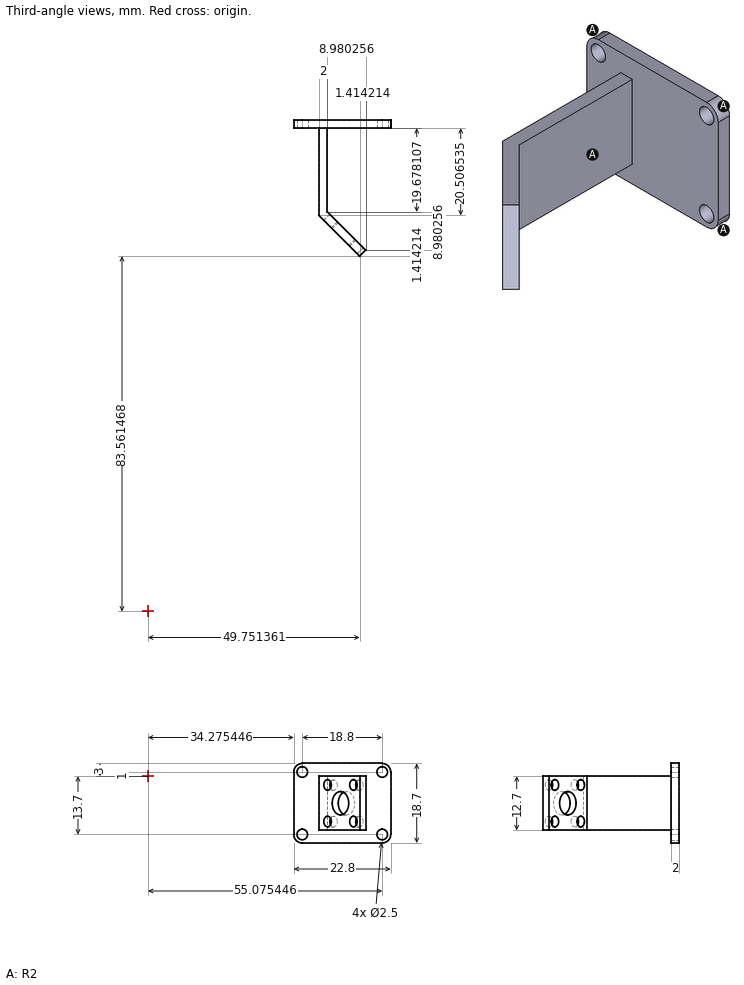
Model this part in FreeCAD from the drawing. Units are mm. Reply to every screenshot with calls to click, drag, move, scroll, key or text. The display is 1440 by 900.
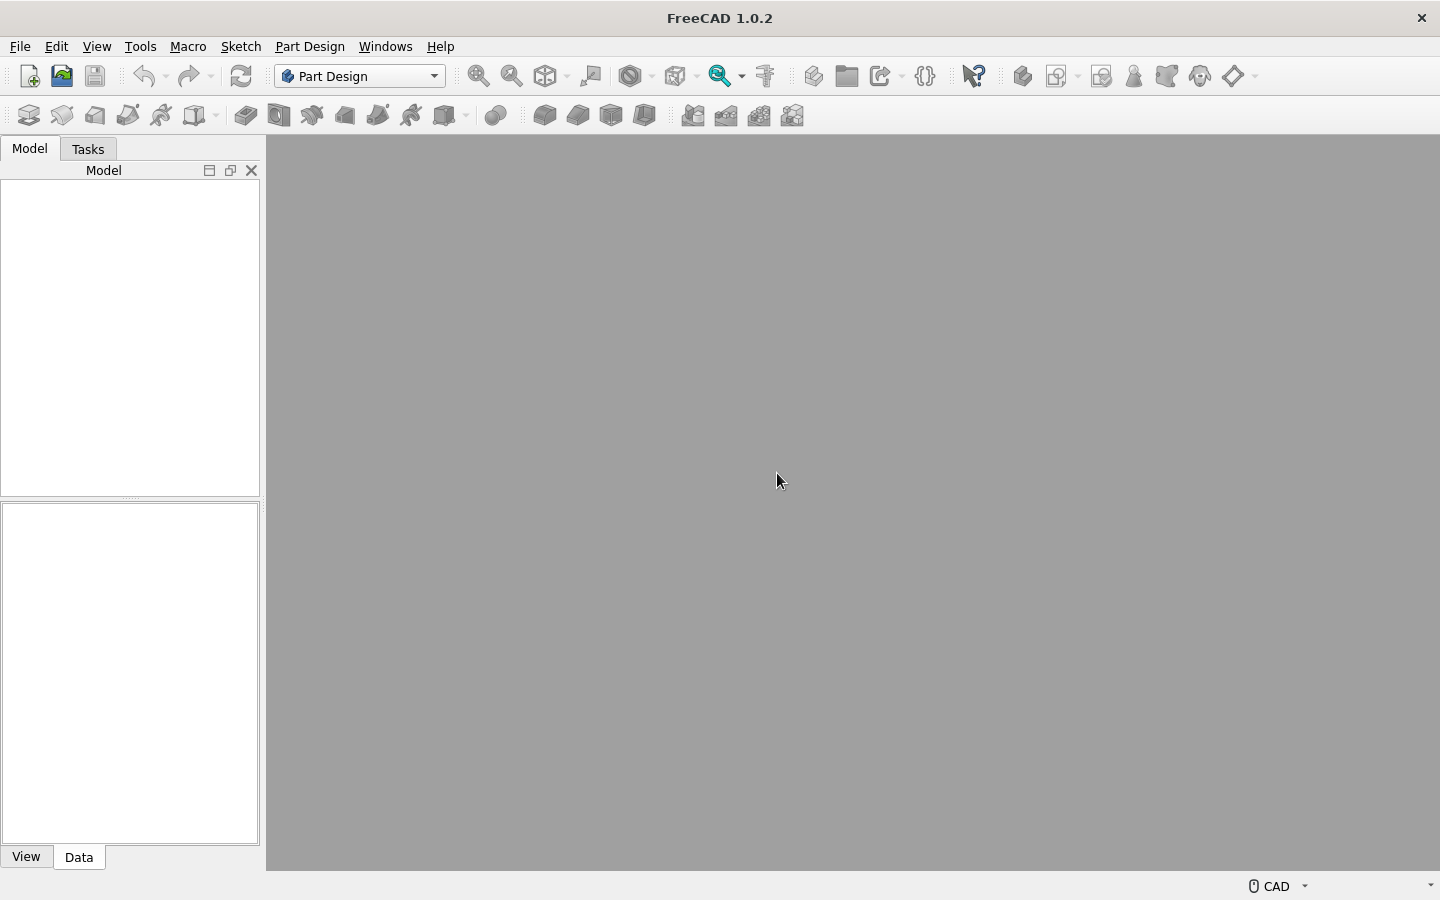
click(29, 76)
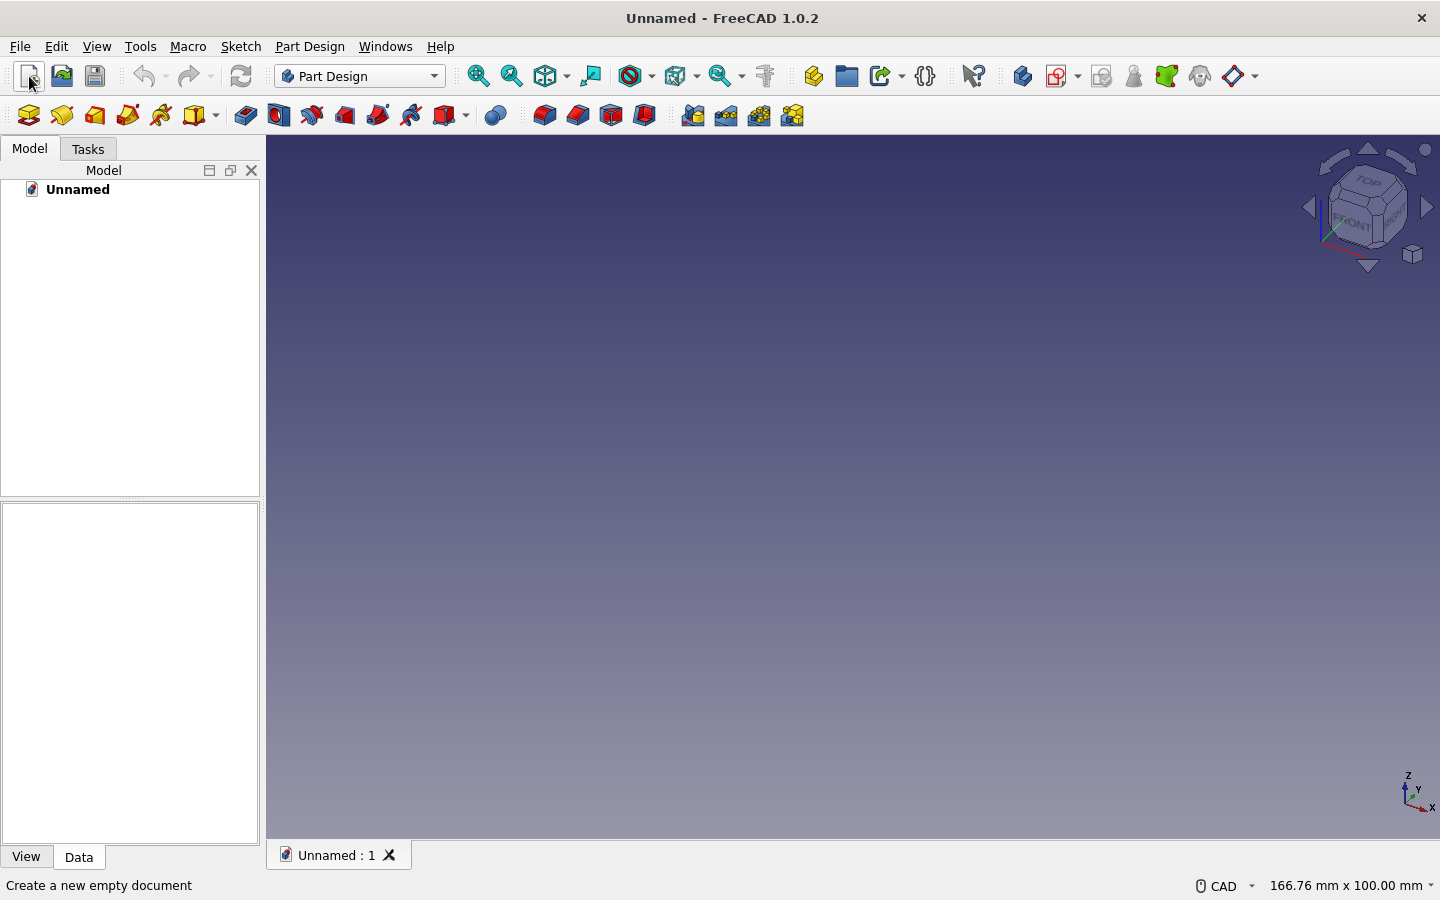
click(1056, 76)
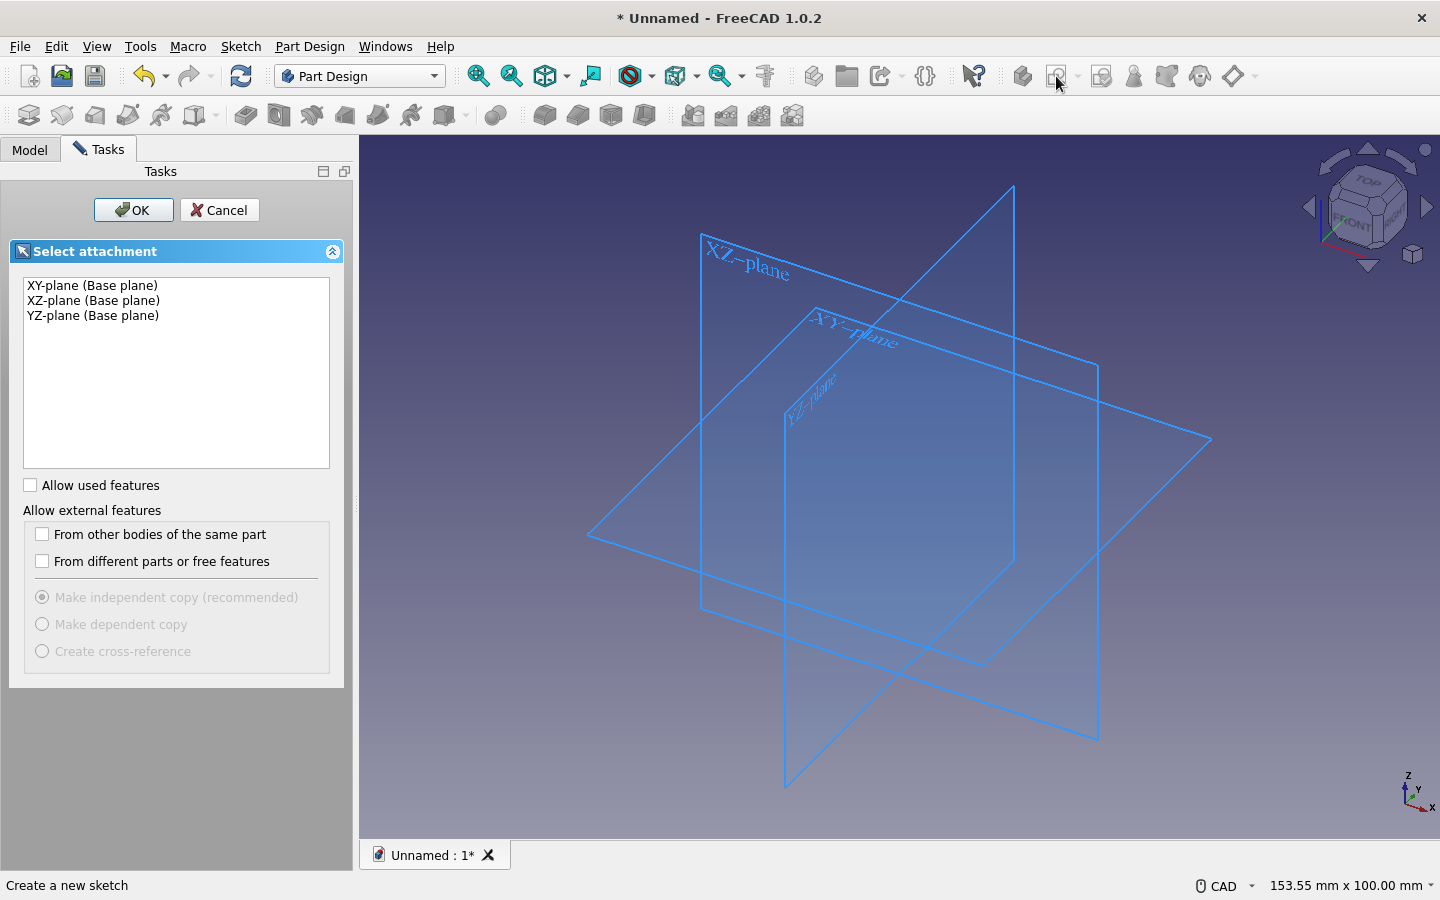
click(84, 286)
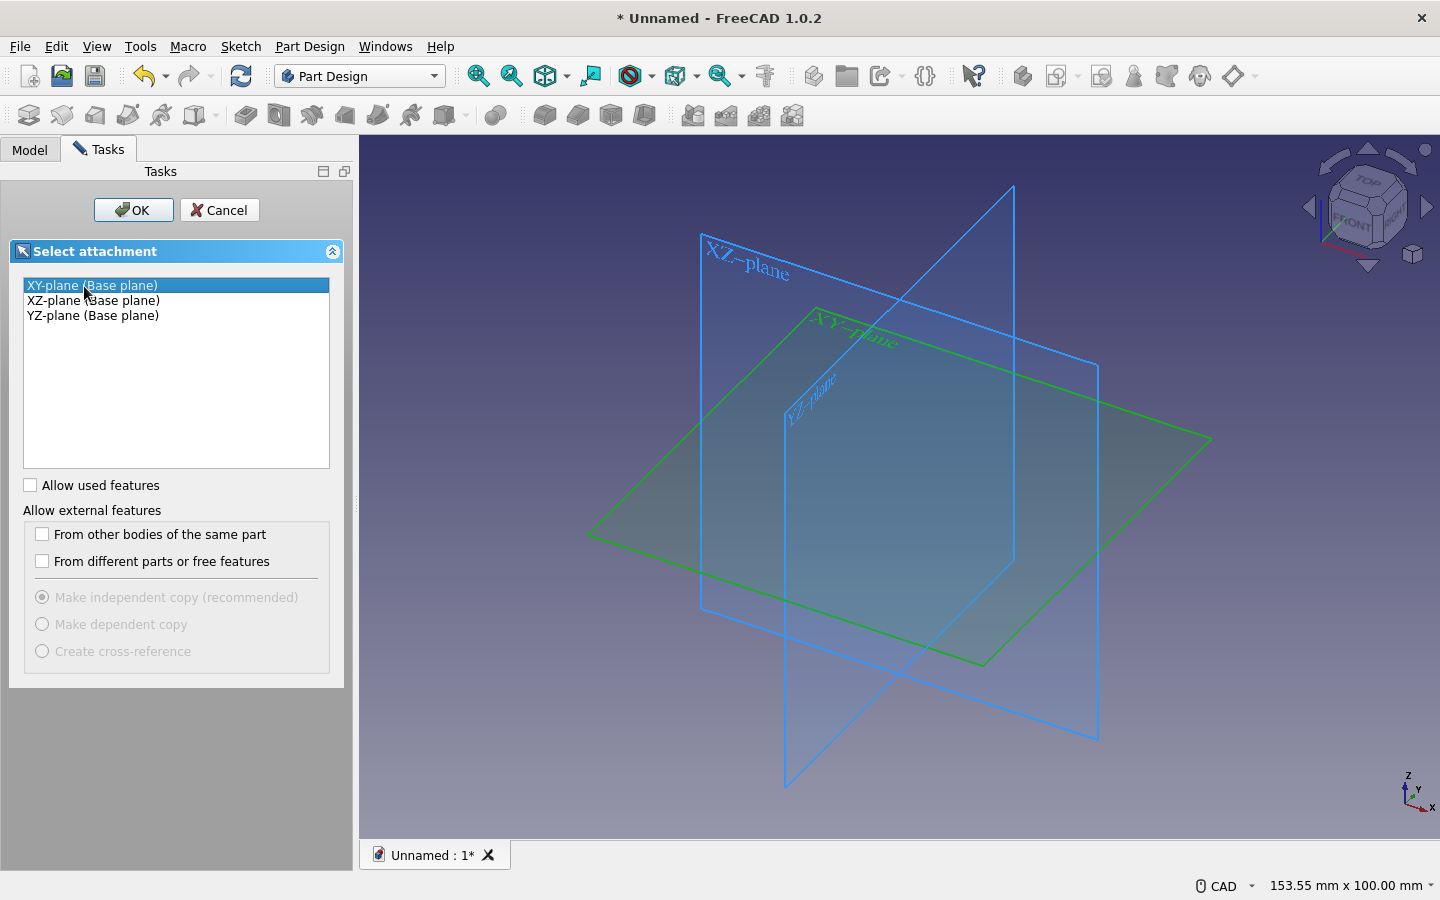
click(134, 210)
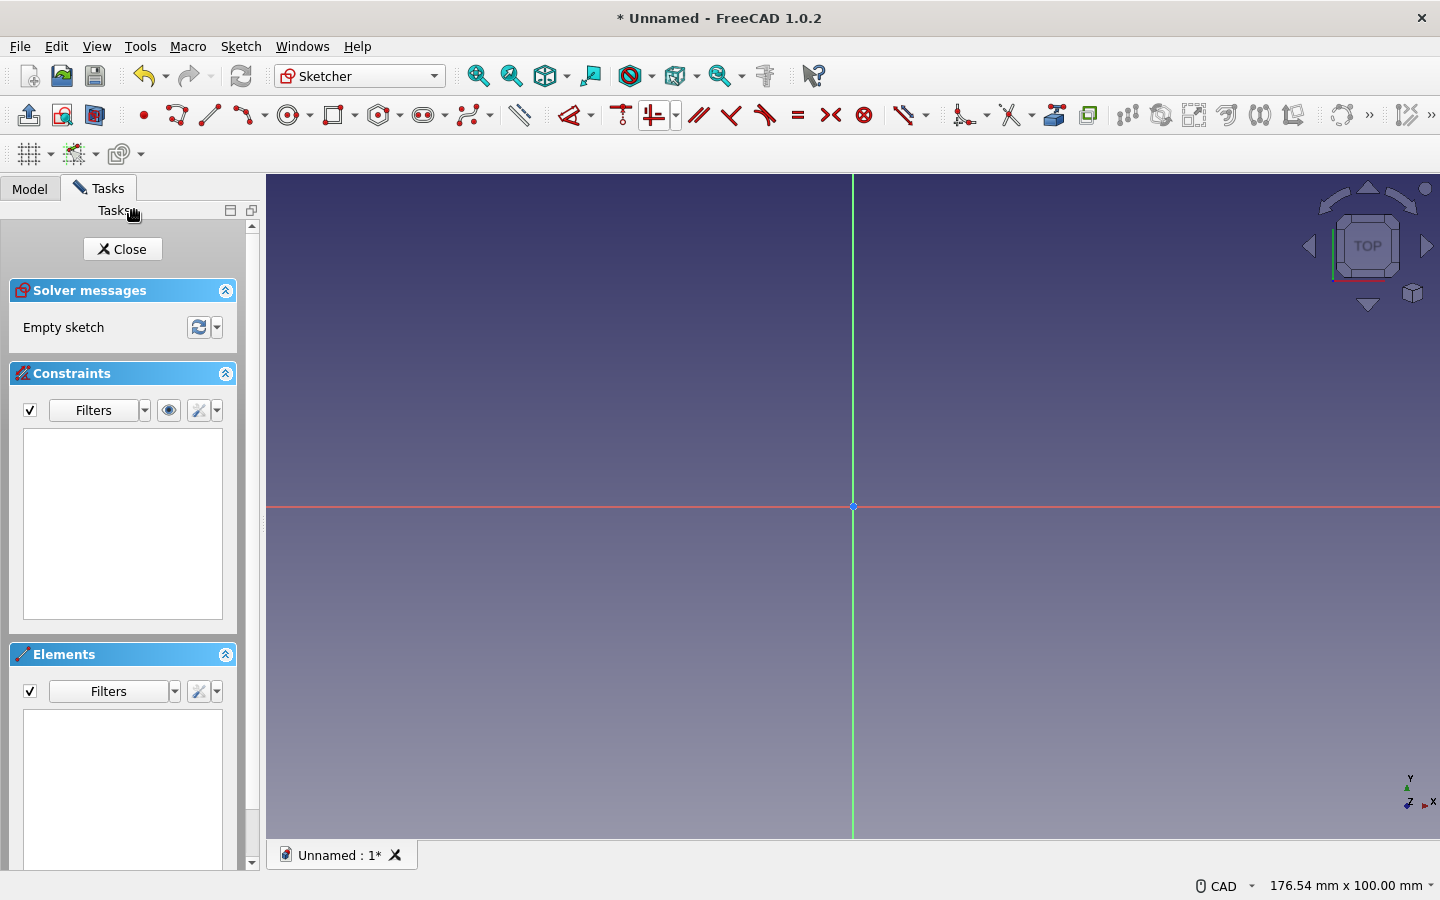
scroll(784, 506, down, 5)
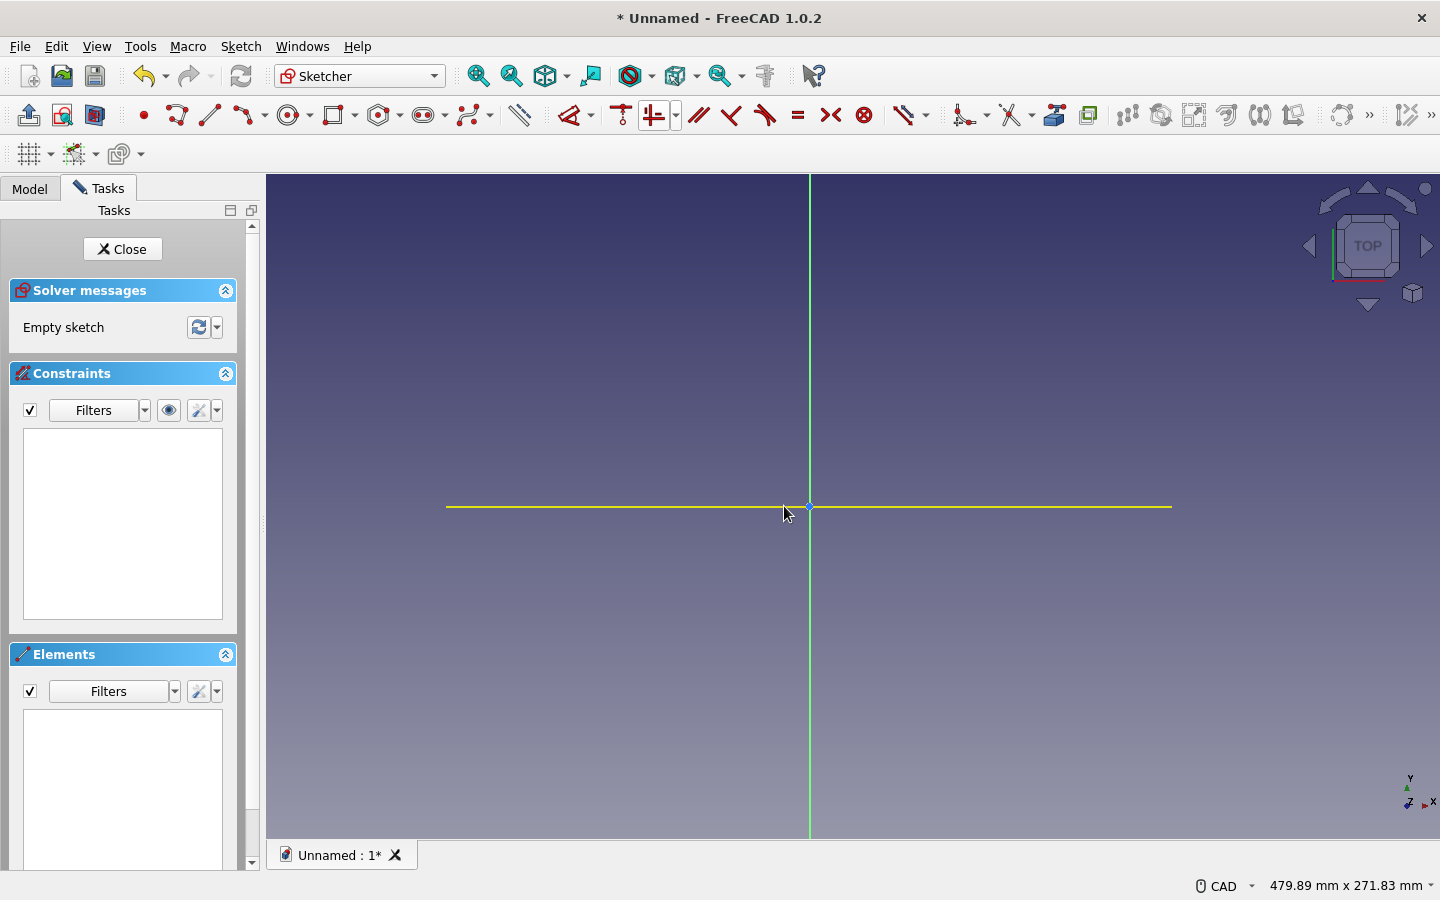
scroll(949, 218, up, 9)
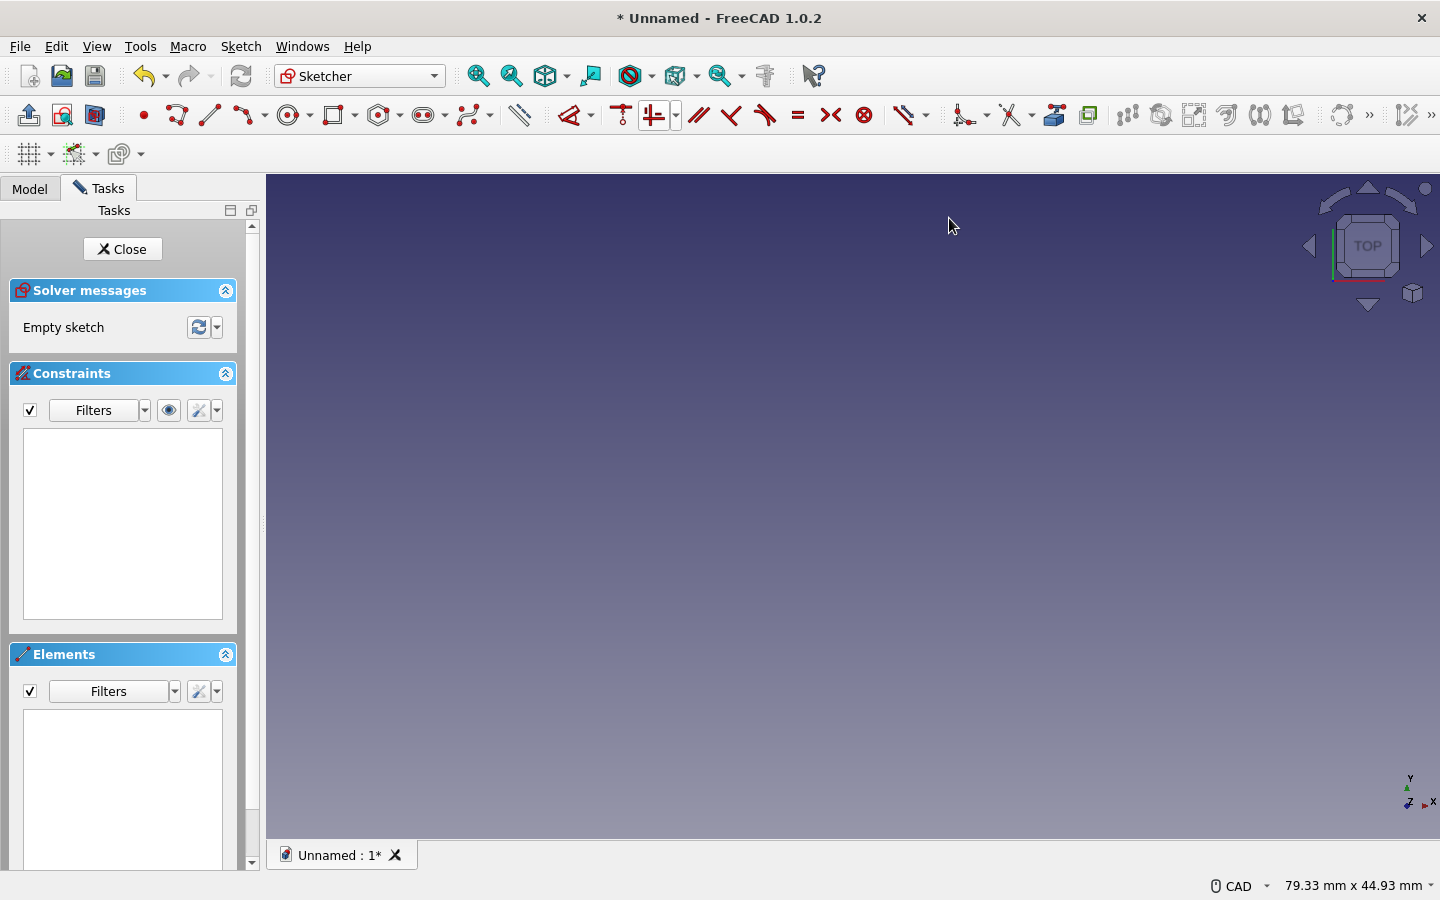
key(g)
key(m)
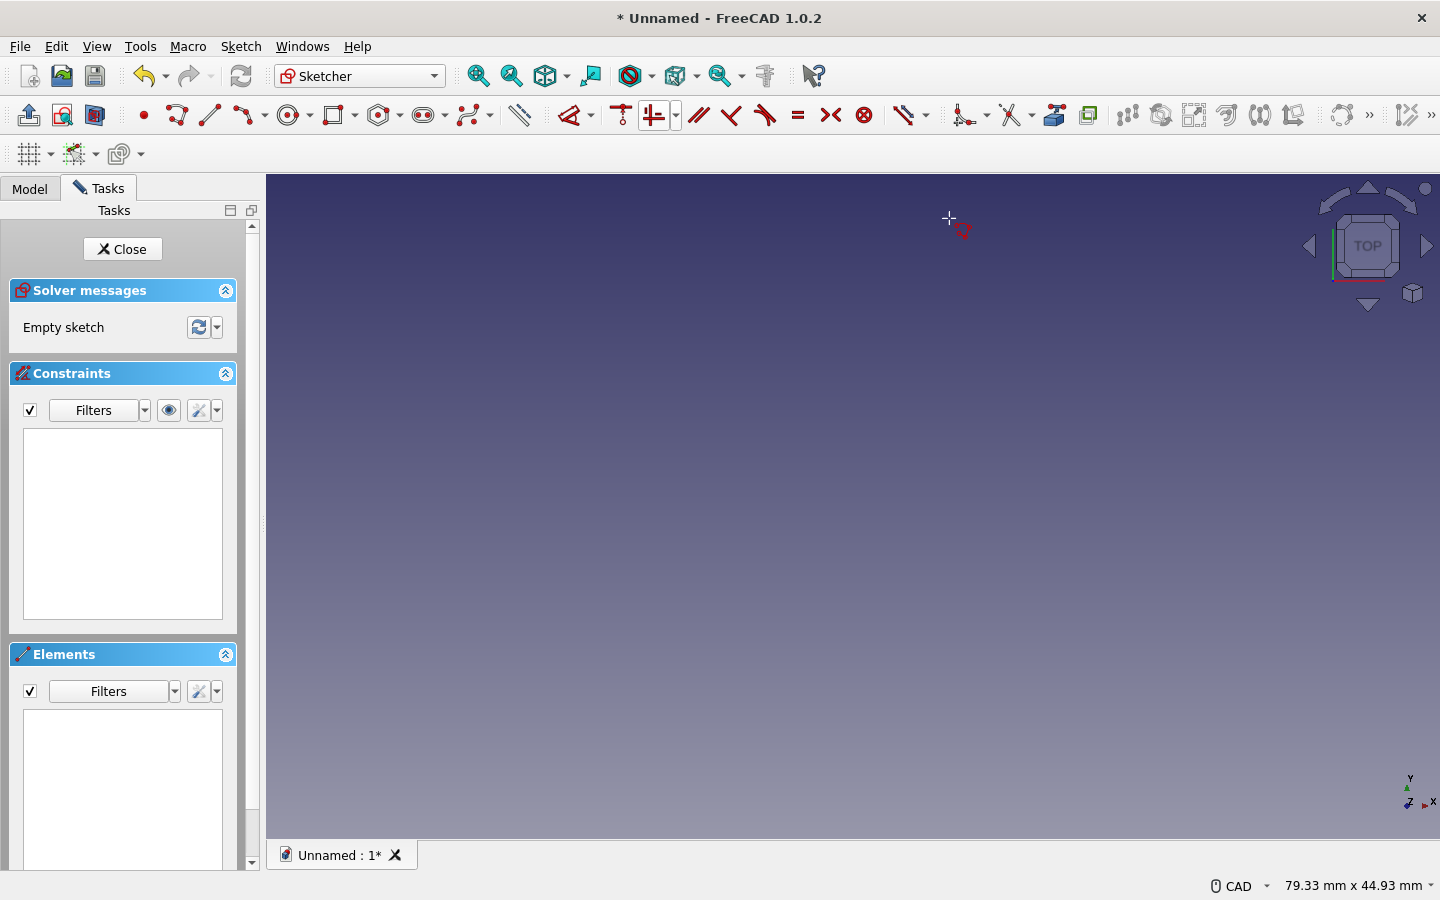
click(839, 726)
click(860, 705)
click(727, 572)
click(727, 281)
click(698, 281)
click(698, 585)
click(839, 727)
key(Escape)
key(Escape)